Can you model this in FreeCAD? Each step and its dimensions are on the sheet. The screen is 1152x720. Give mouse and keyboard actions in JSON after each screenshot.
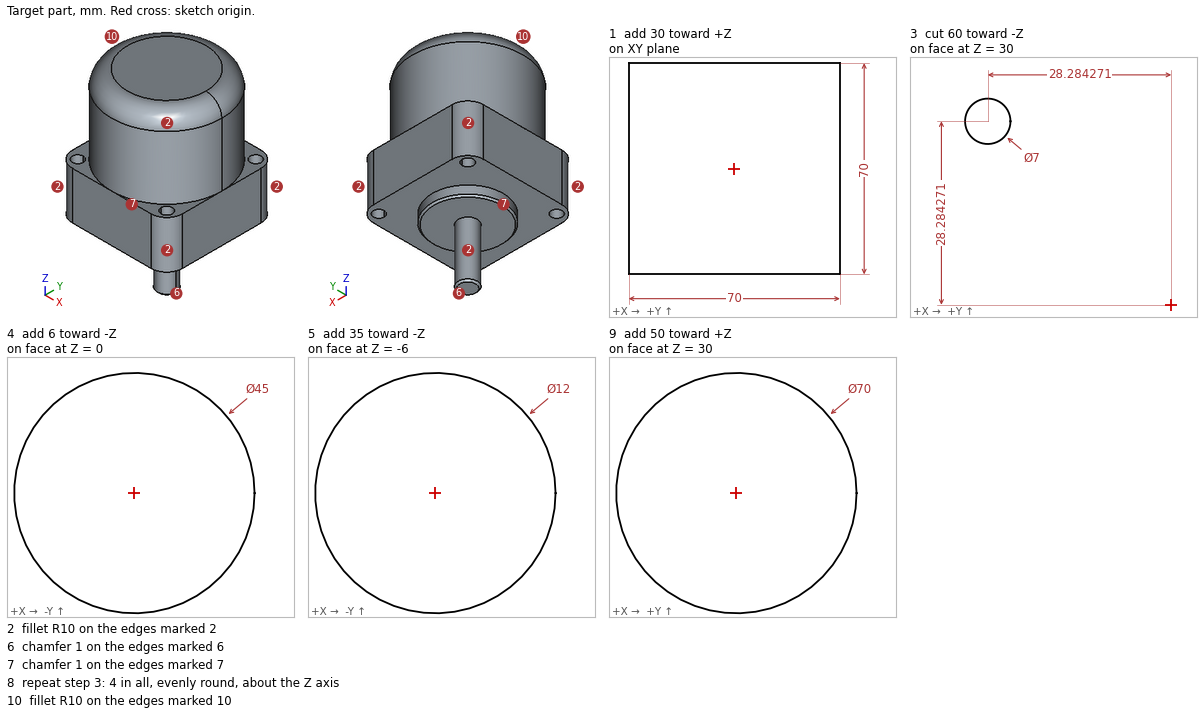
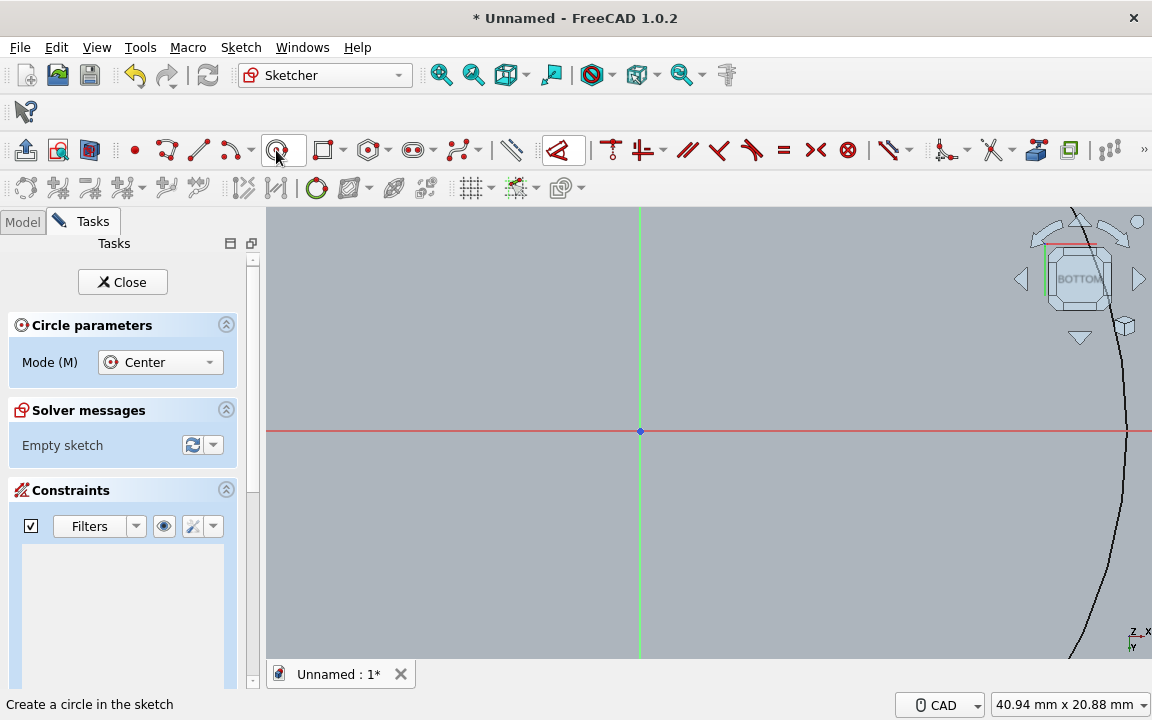
{"action": "left_click", "coordinate": [640, 431]}
{"action": "mouse_move", "coordinate": [732, 339]}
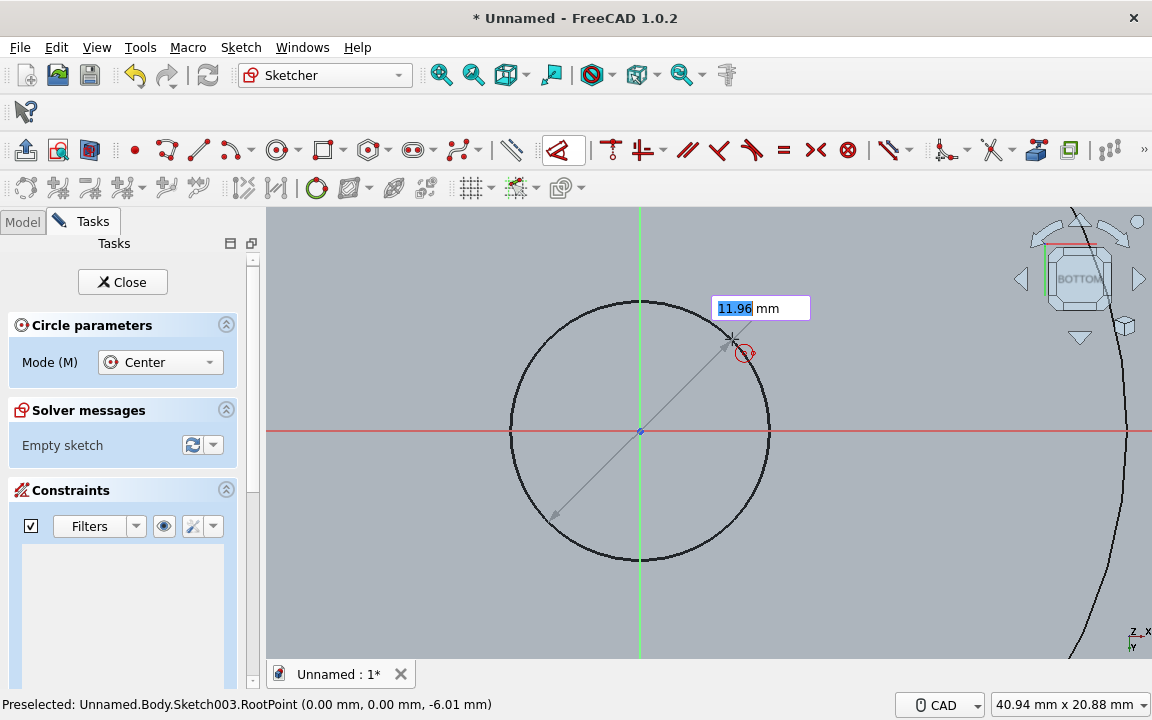
{"action": "type", "text": "12"}
{"action": "key", "text": "Return"}
{"action": "key", "text": "Escape"}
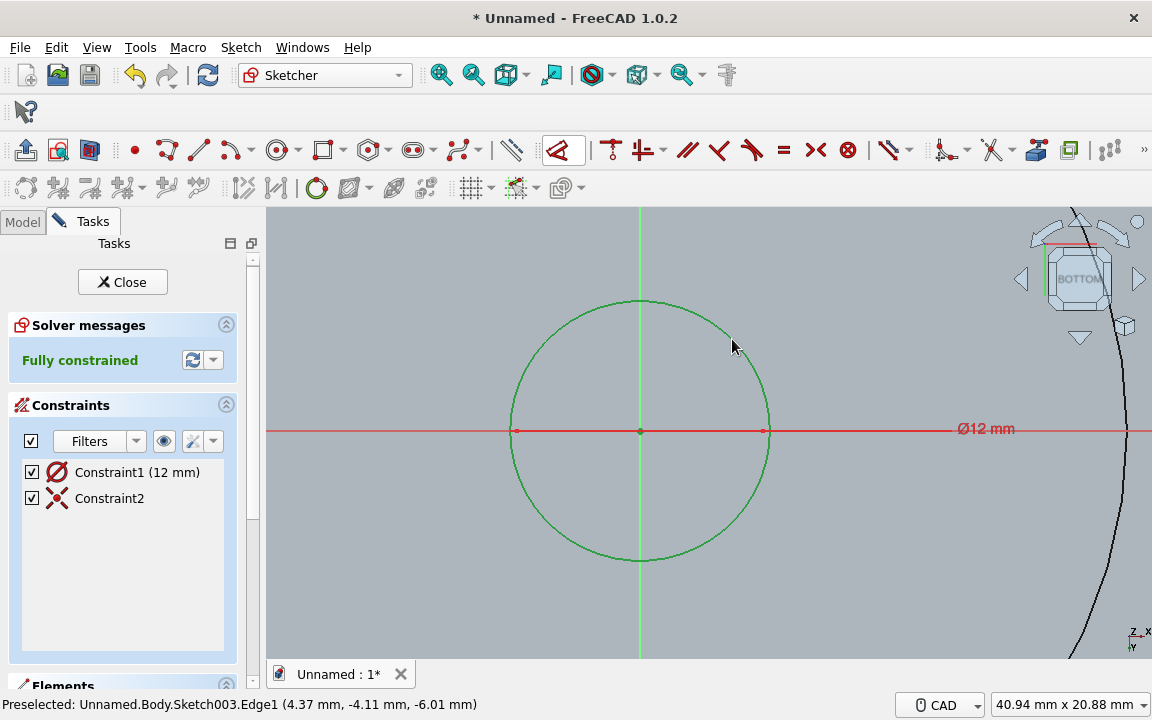
{"action": "left_click", "coordinate": [123, 282]}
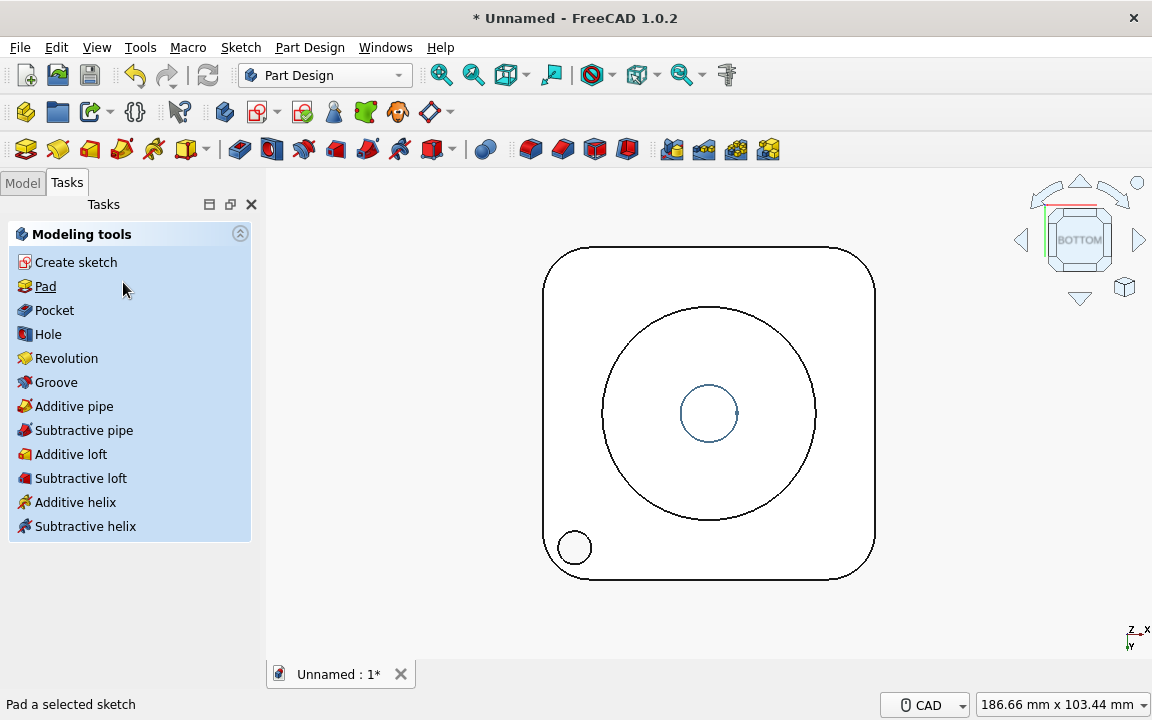
{"action": "left_click", "coordinate": [26, 150]}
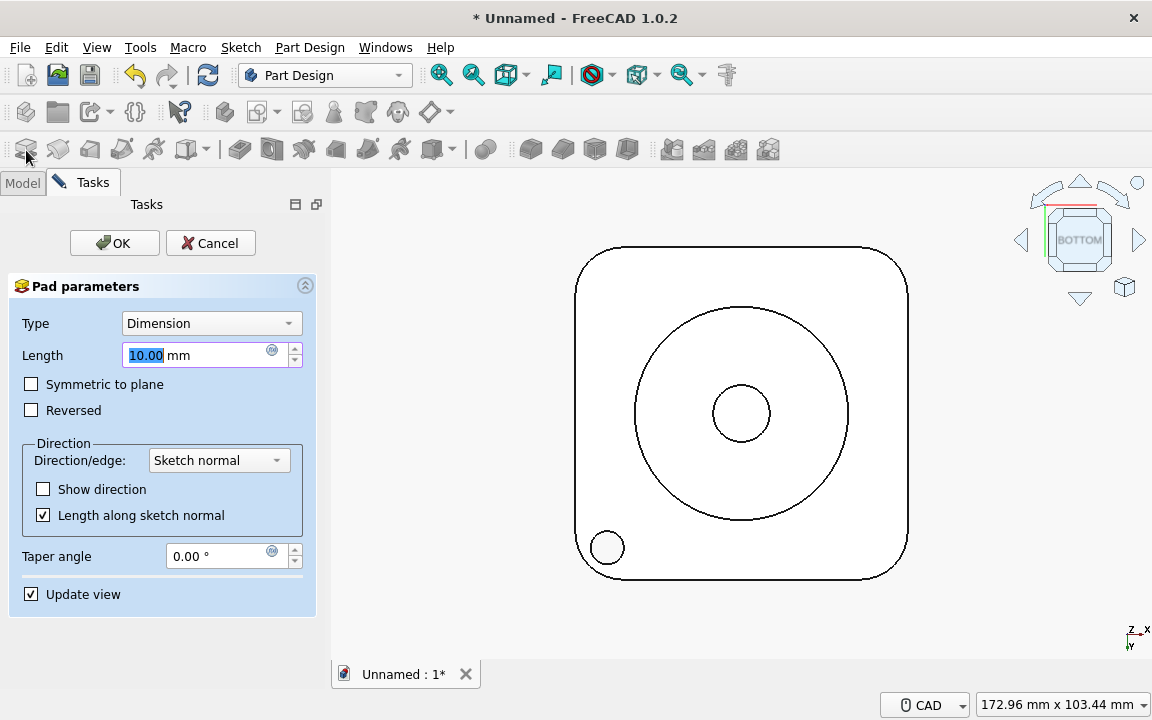
{"action": "type", "text": "35"}
{"action": "key", "text": "Tab"}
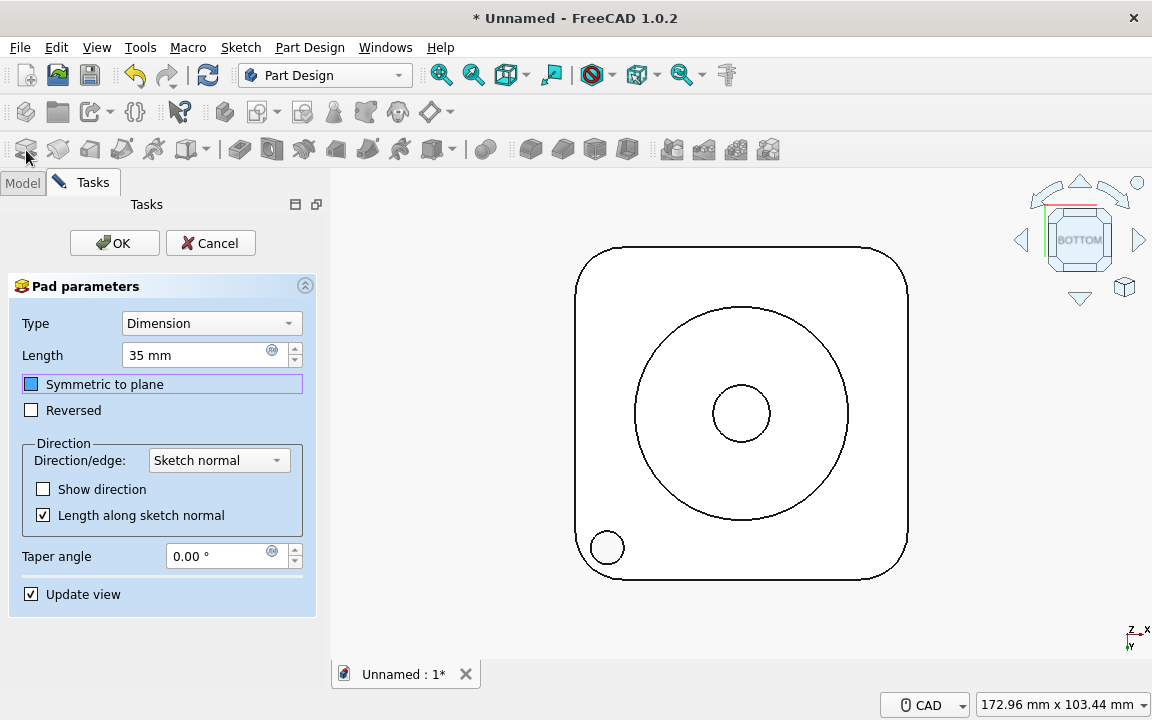
{"action": "left_click", "coordinate": [115, 243]}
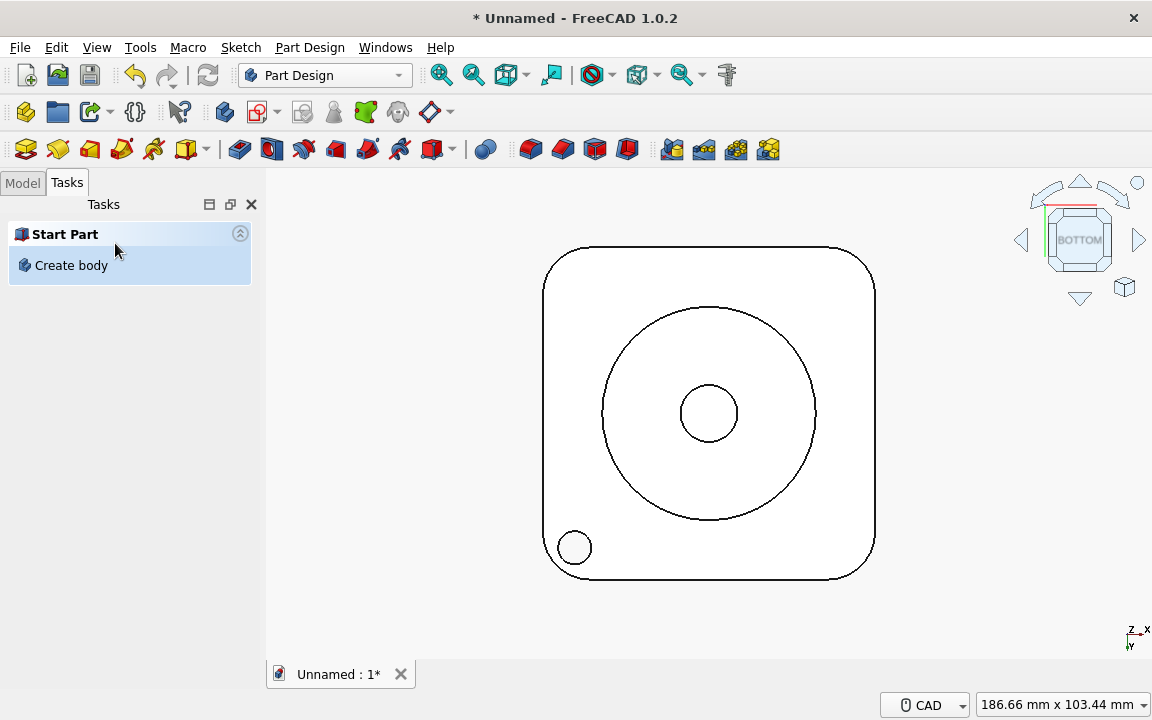
{"action": "left_click", "coordinate": [681, 413]}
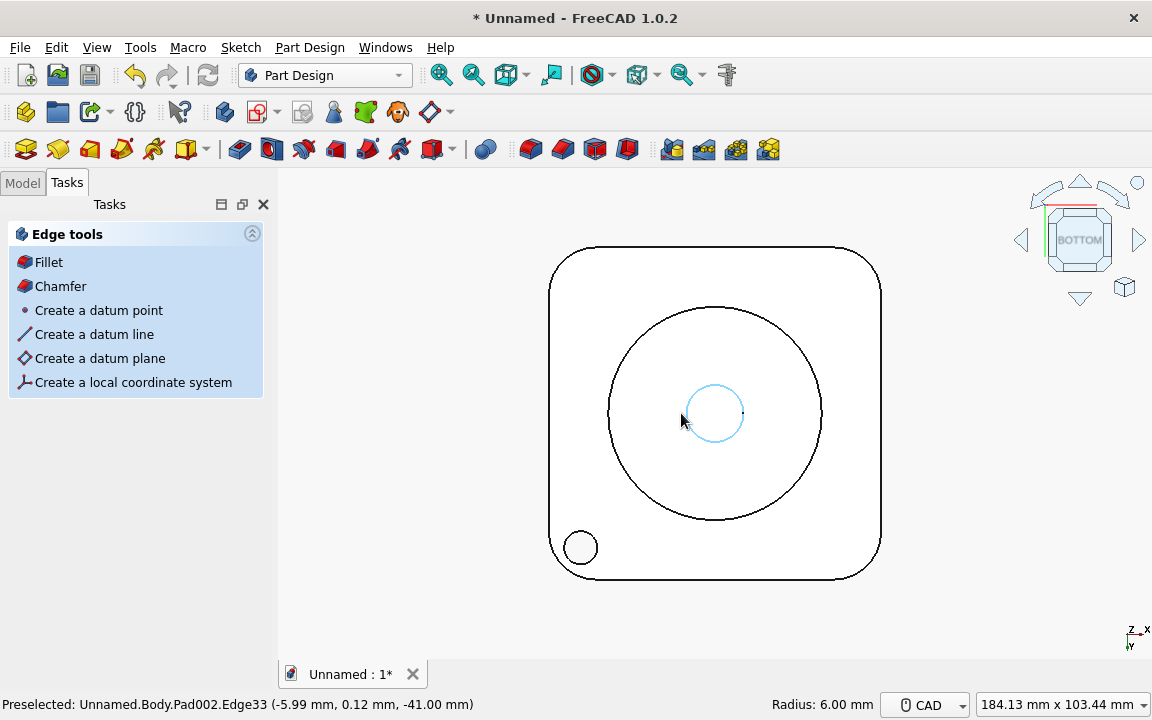
{"action": "left_click", "coordinate": [564, 150]}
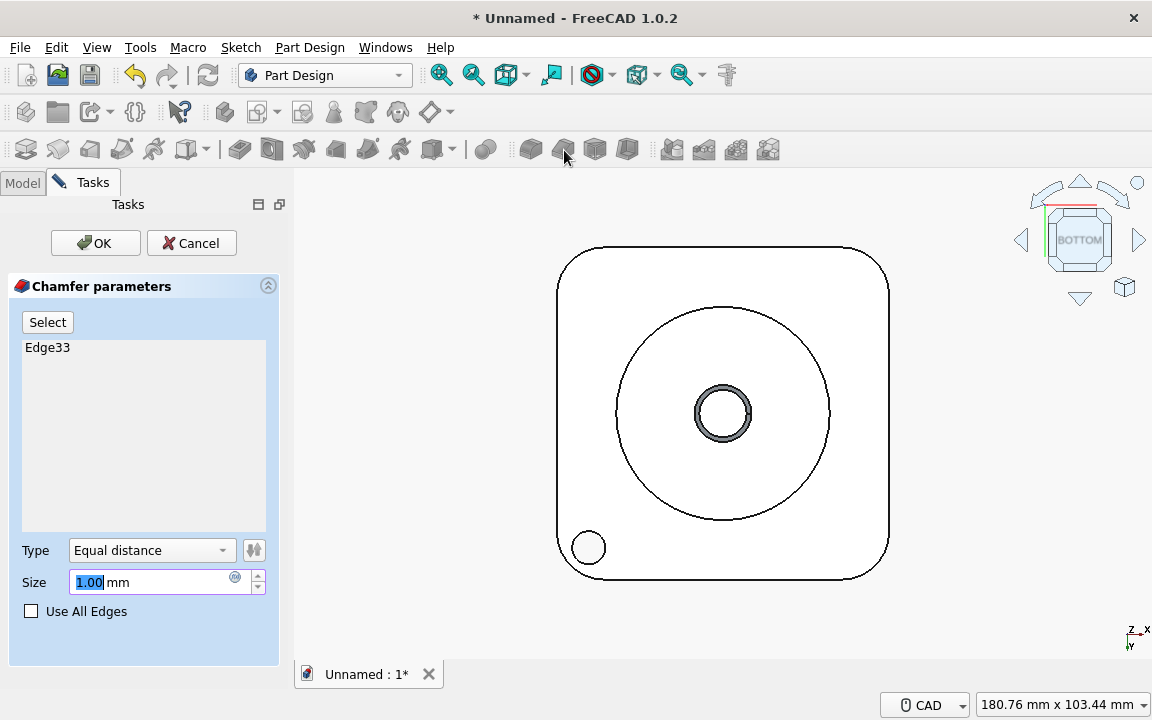
{"action": "type", "text": "1"}
{"action": "key", "text": "Tab"}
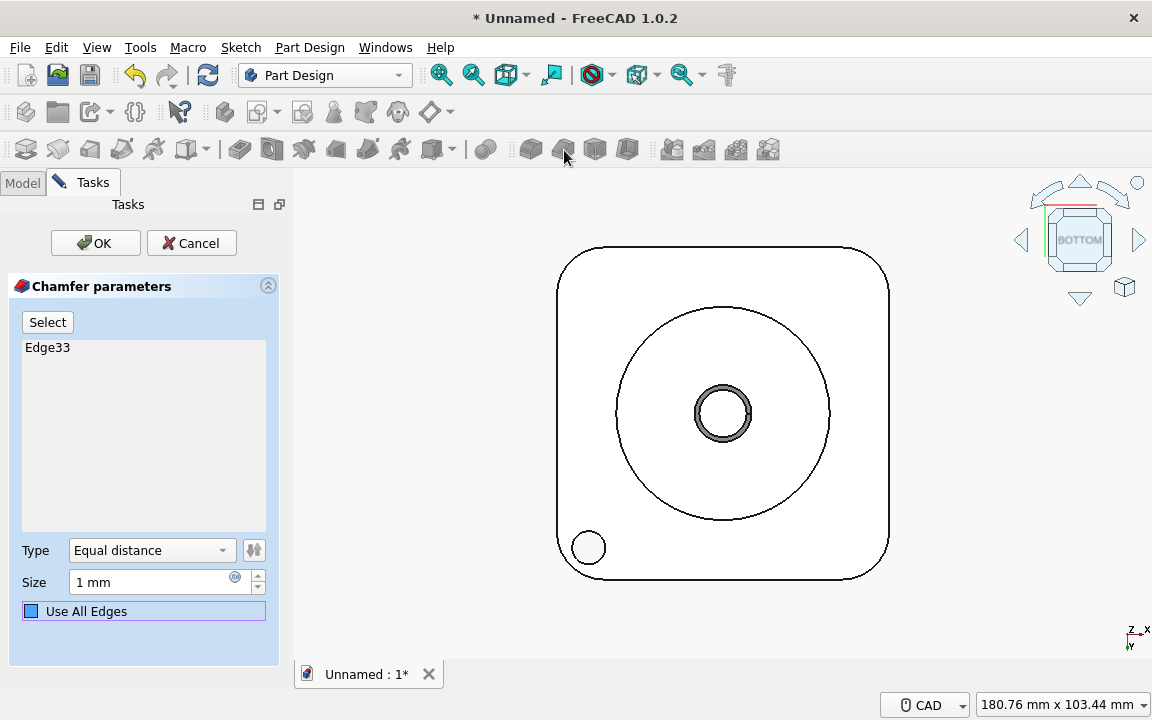
{"action": "left_click", "coordinate": [96, 243]}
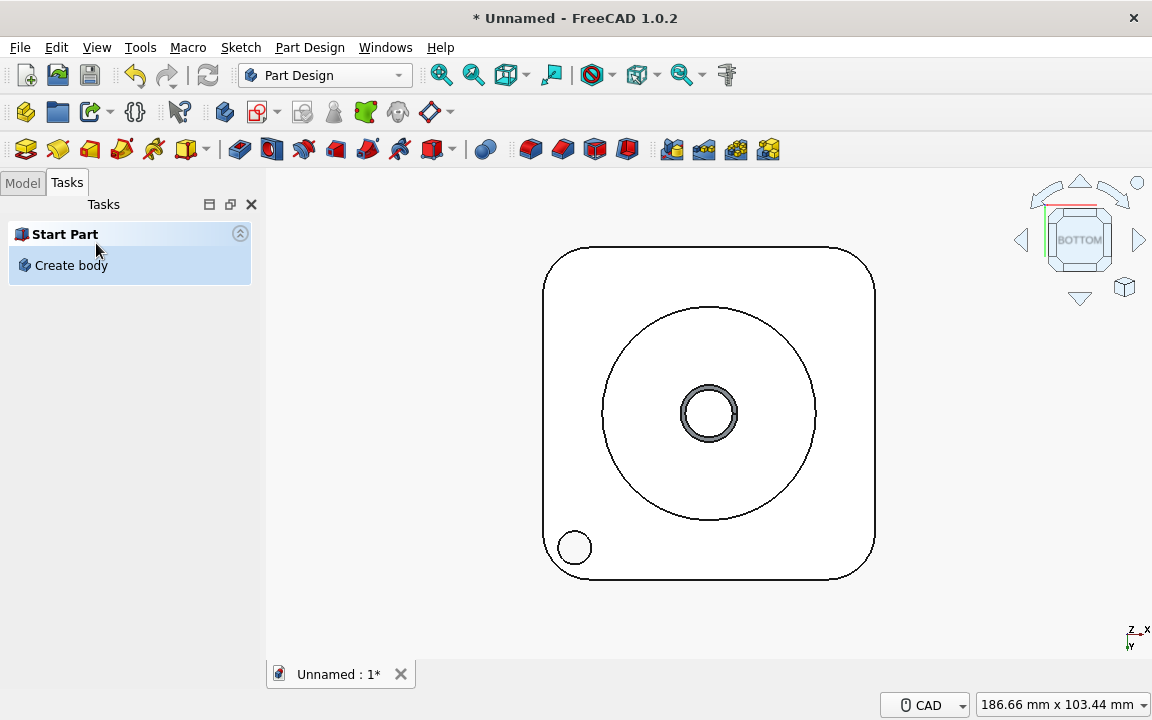
{"action": "left_click", "coordinate": [602, 413]}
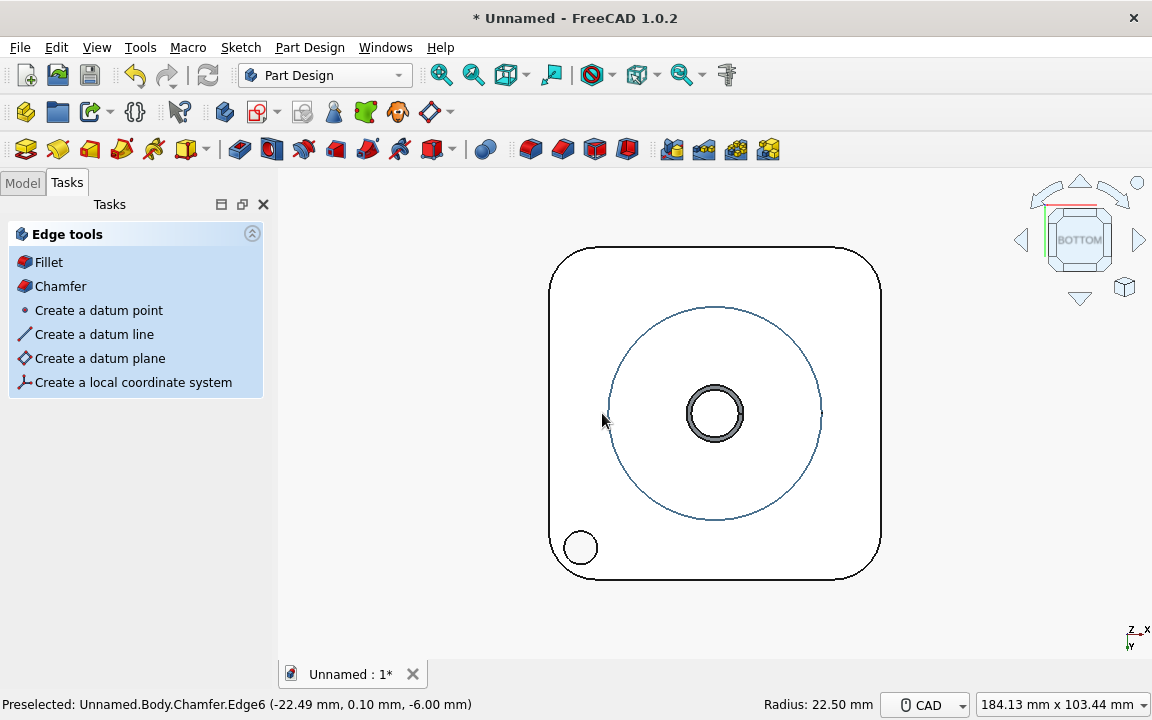
{"action": "left_click", "coordinate": [564, 150]}